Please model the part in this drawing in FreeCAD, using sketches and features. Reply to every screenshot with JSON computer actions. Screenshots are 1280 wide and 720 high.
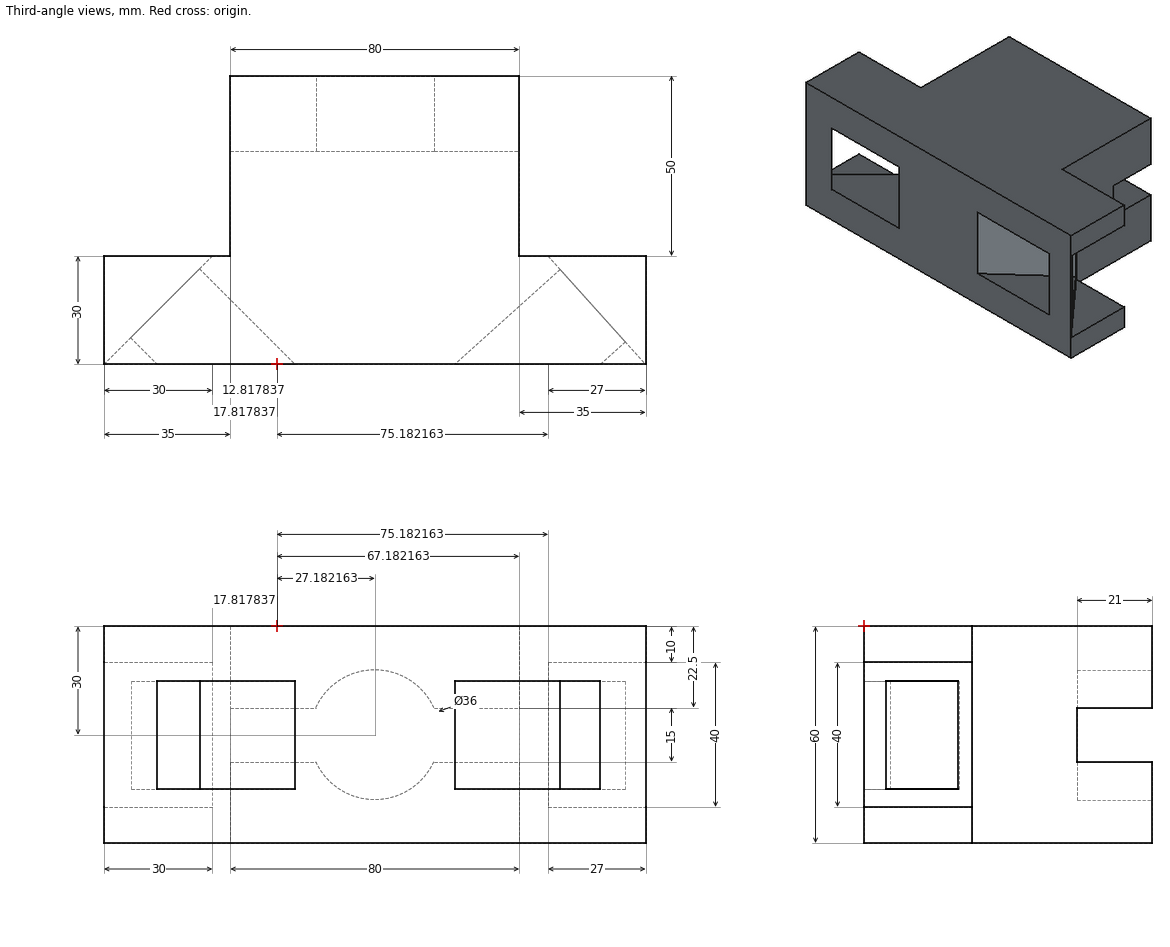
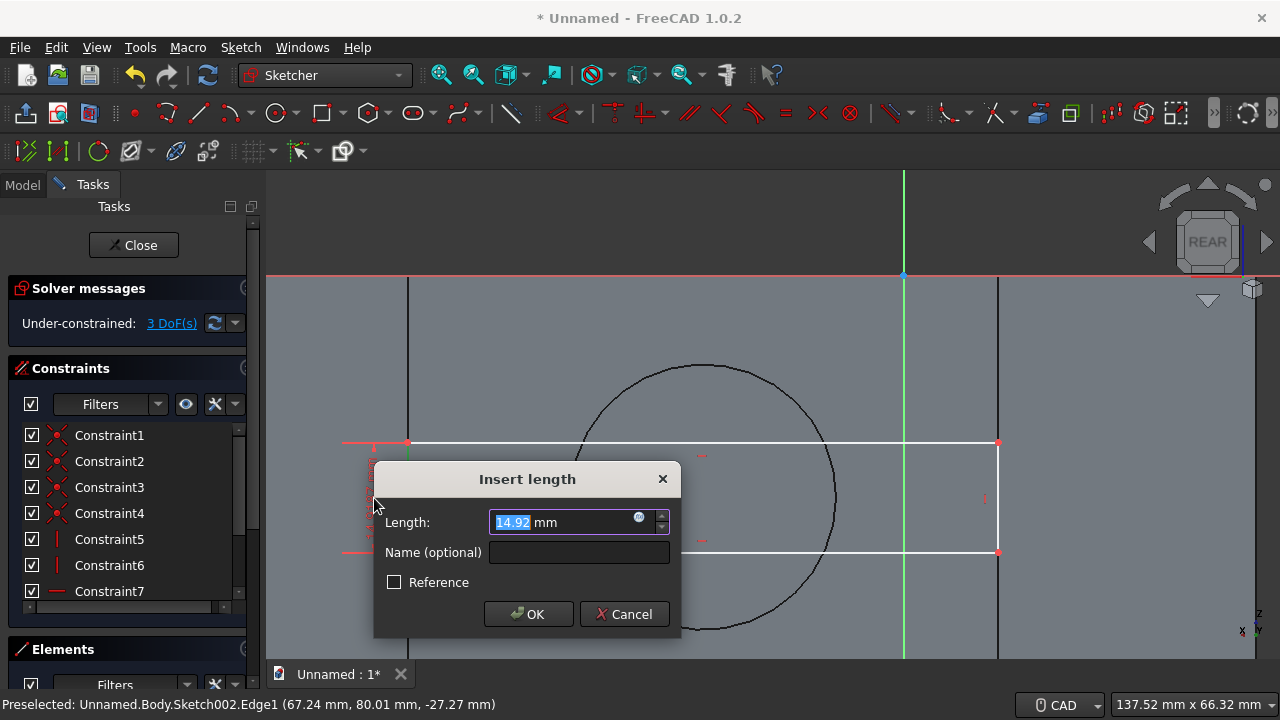
{"action": "type", "text": "15"}
{"action": "key", "text": "Return"}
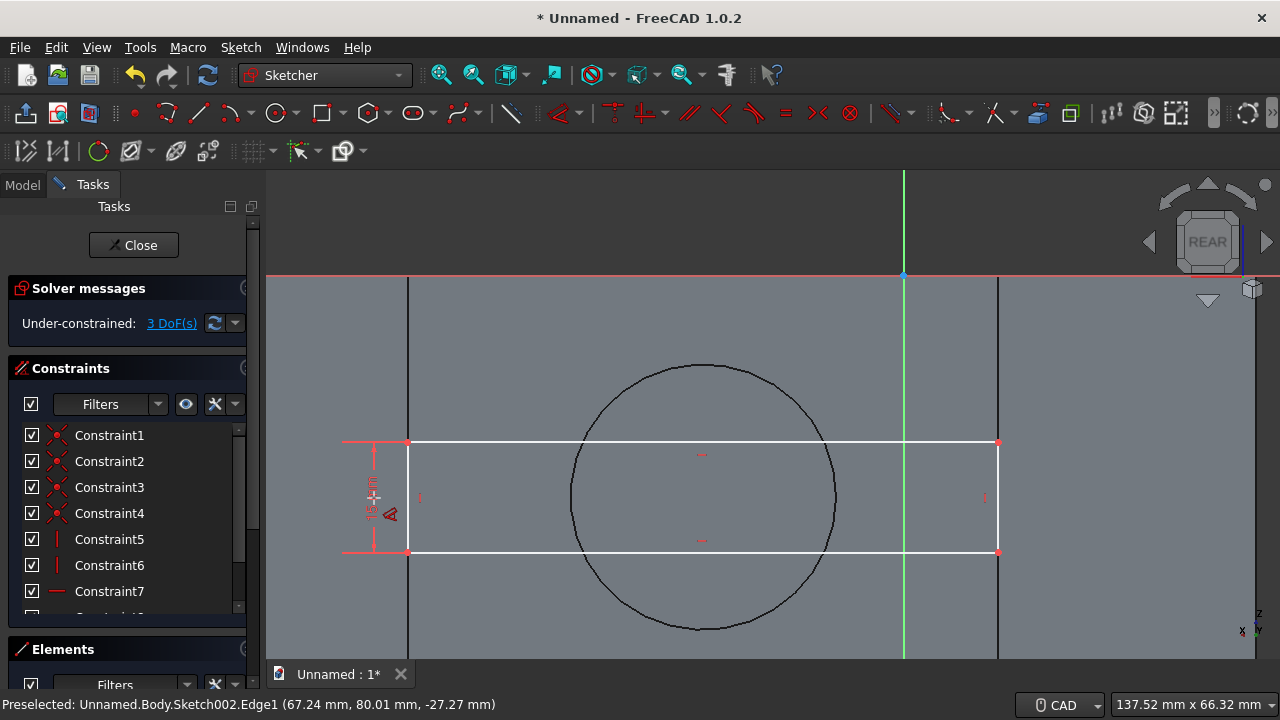
{"action": "left_click", "coordinate": [585, 553]}
{"action": "left_click", "coordinate": [703, 587]}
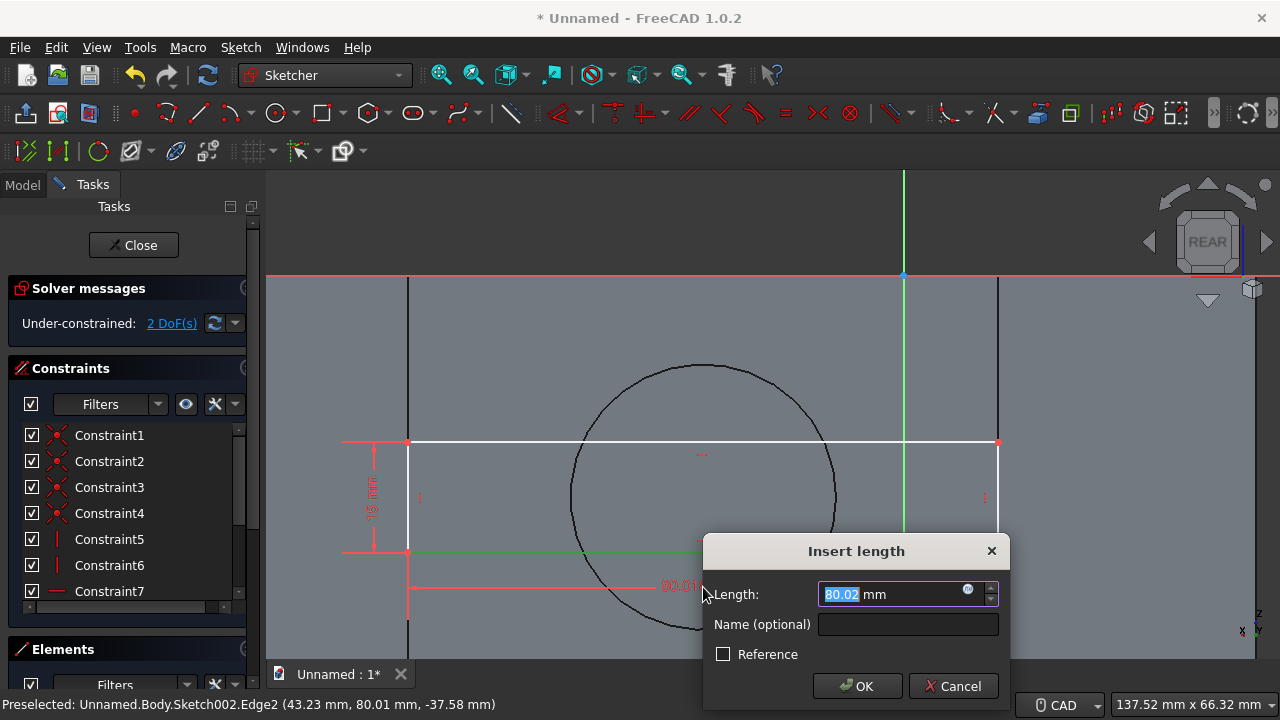
{"action": "type", "text": "80"}
{"action": "key", "text": "Return"}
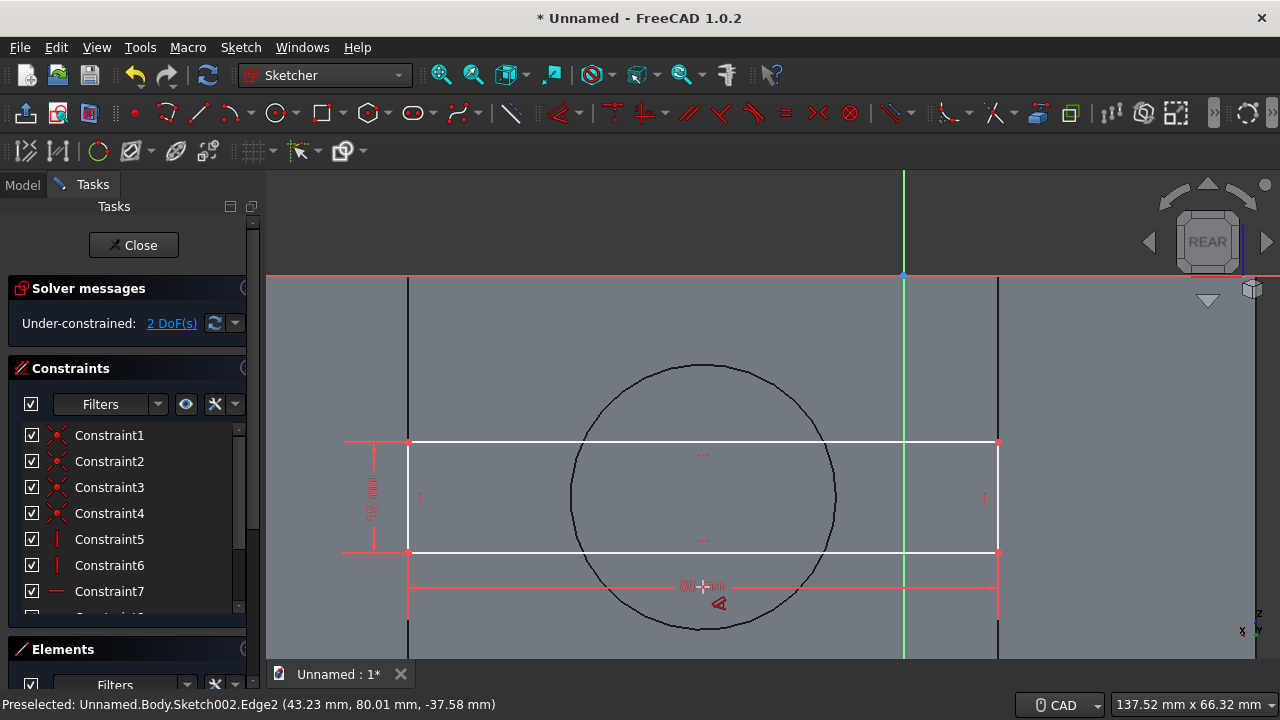
{"action": "left_click", "coordinate": [408, 442]}
{"action": "left_click", "coordinate": [374, 359]}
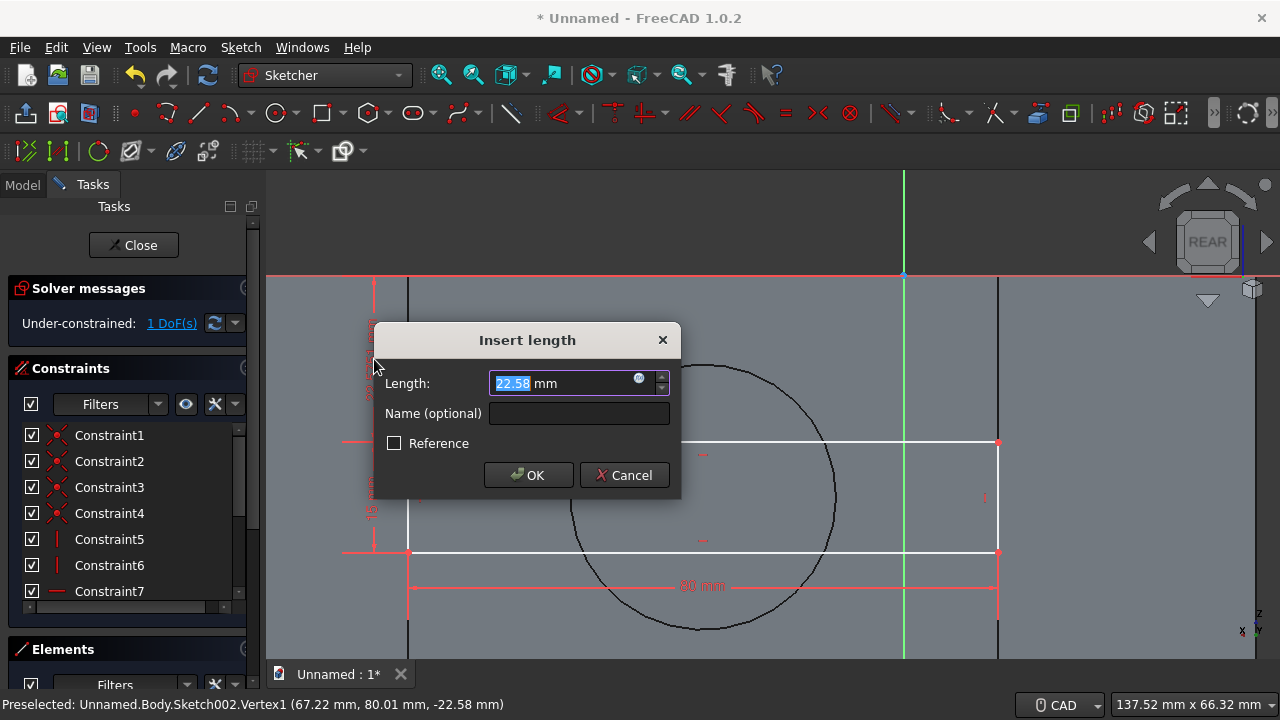
{"action": "type", "text": "22.5"}
{"action": "key", "text": "Return"}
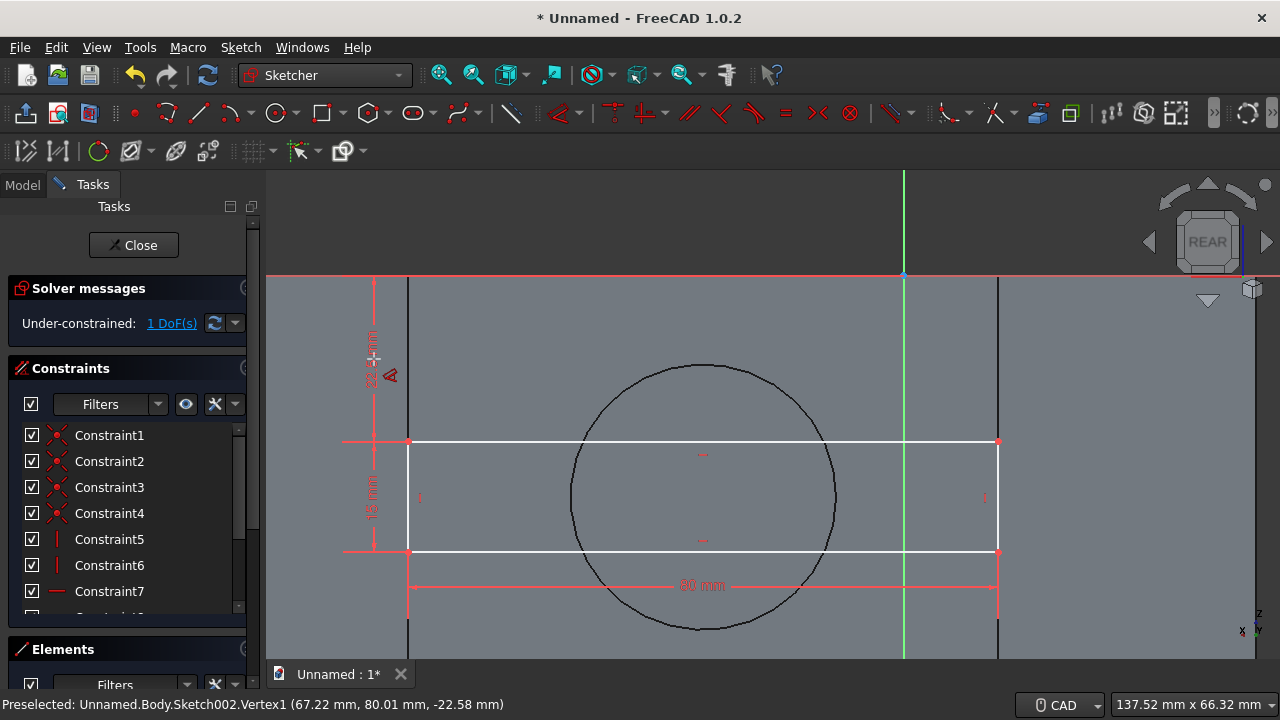
{"action": "left_click", "coordinate": [408, 442]}
{"action": "left_click", "coordinate": [656, 242]}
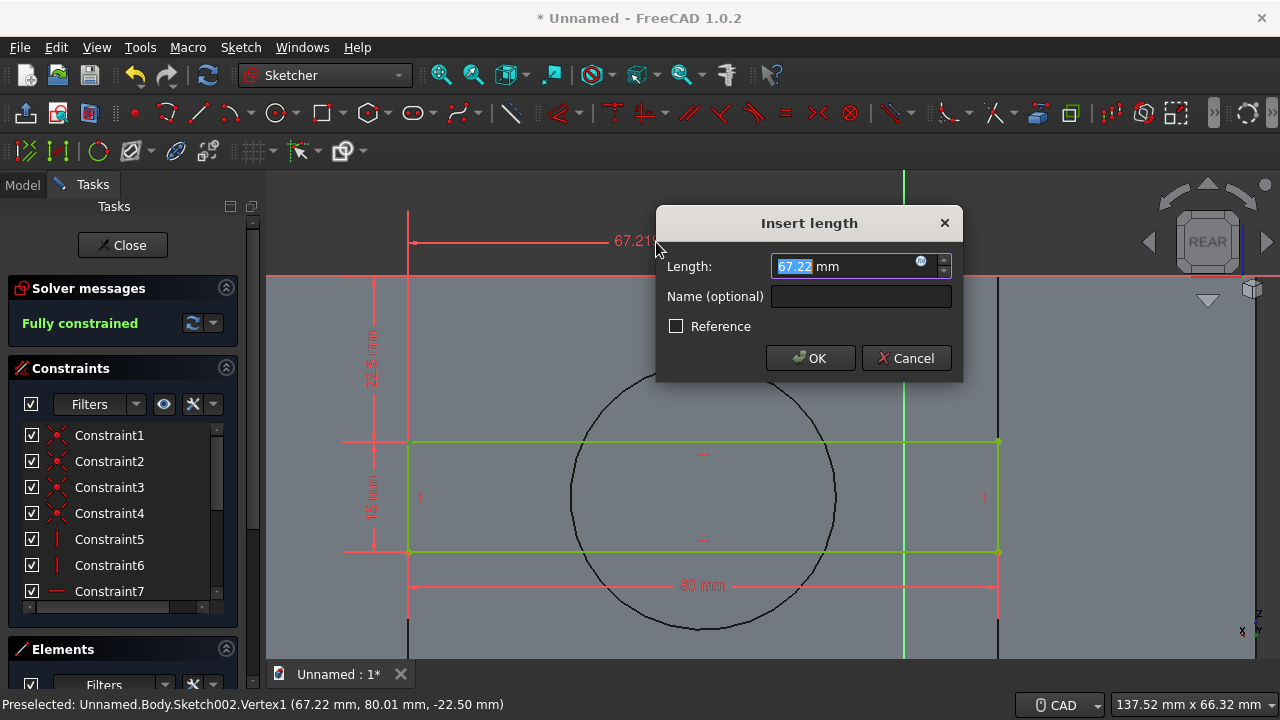
{"action": "type", "text": "67.182163"}
{"action": "key", "text": "Return"}
{"action": "key", "text": "Escape"}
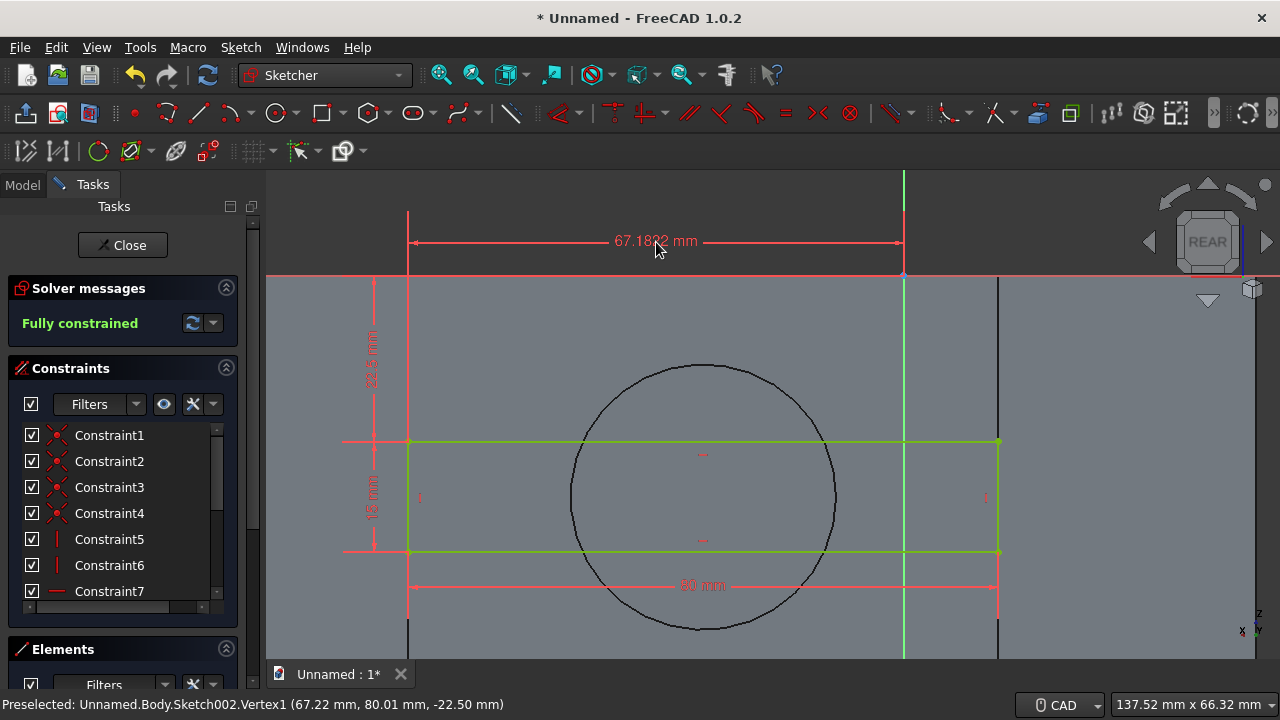
{"action": "left_click", "coordinate": [123, 245]}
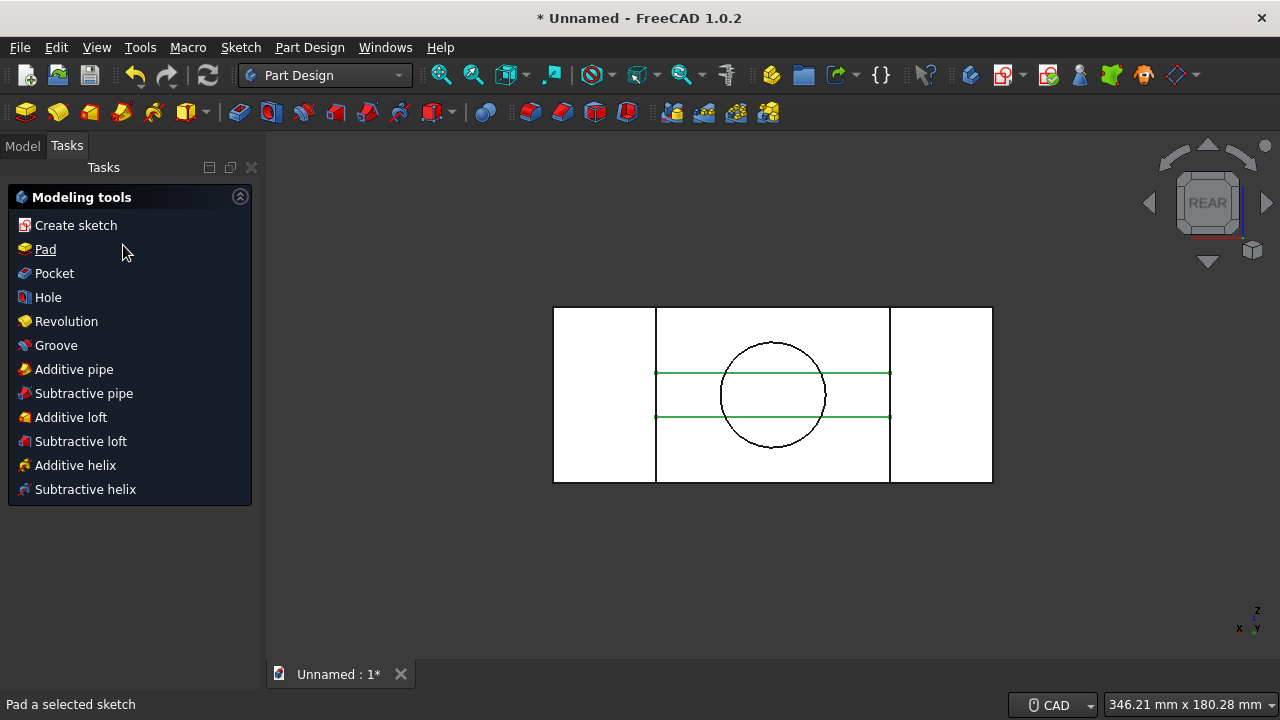
{"action": "left_click", "coordinate": [240, 112]}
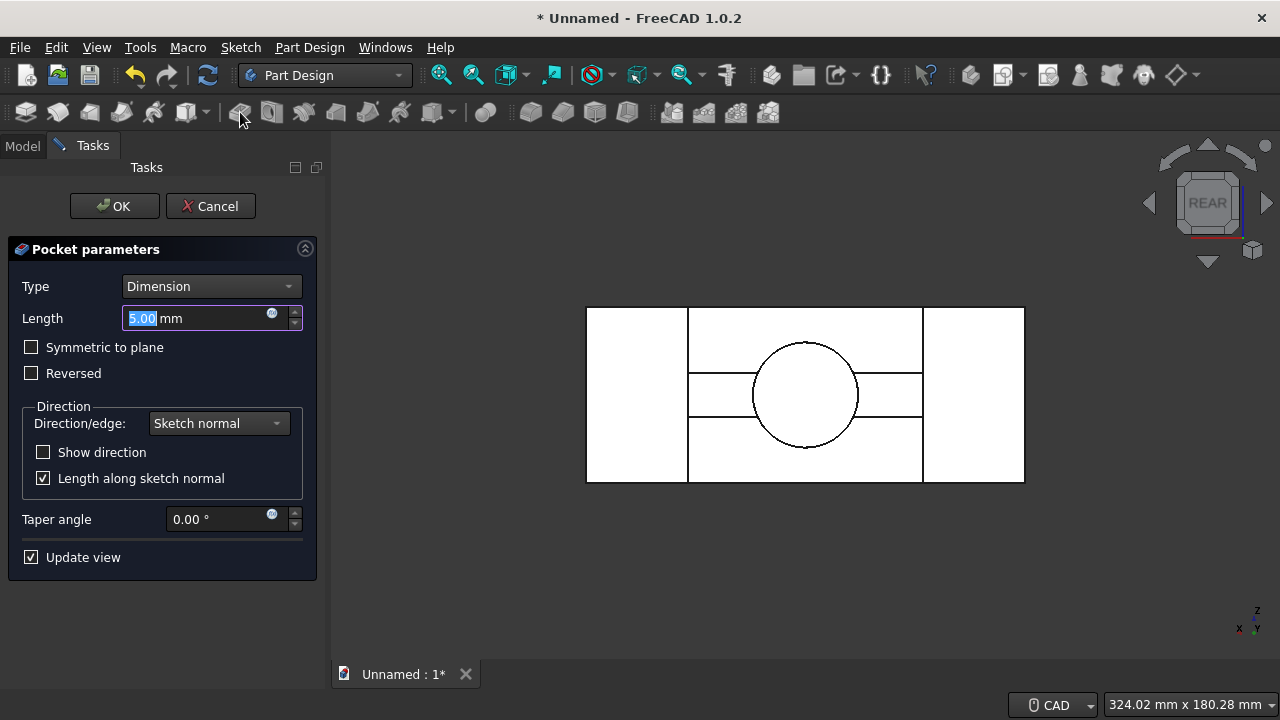
{"action": "type", "text": "21"}
{"action": "key", "text": "Tab"}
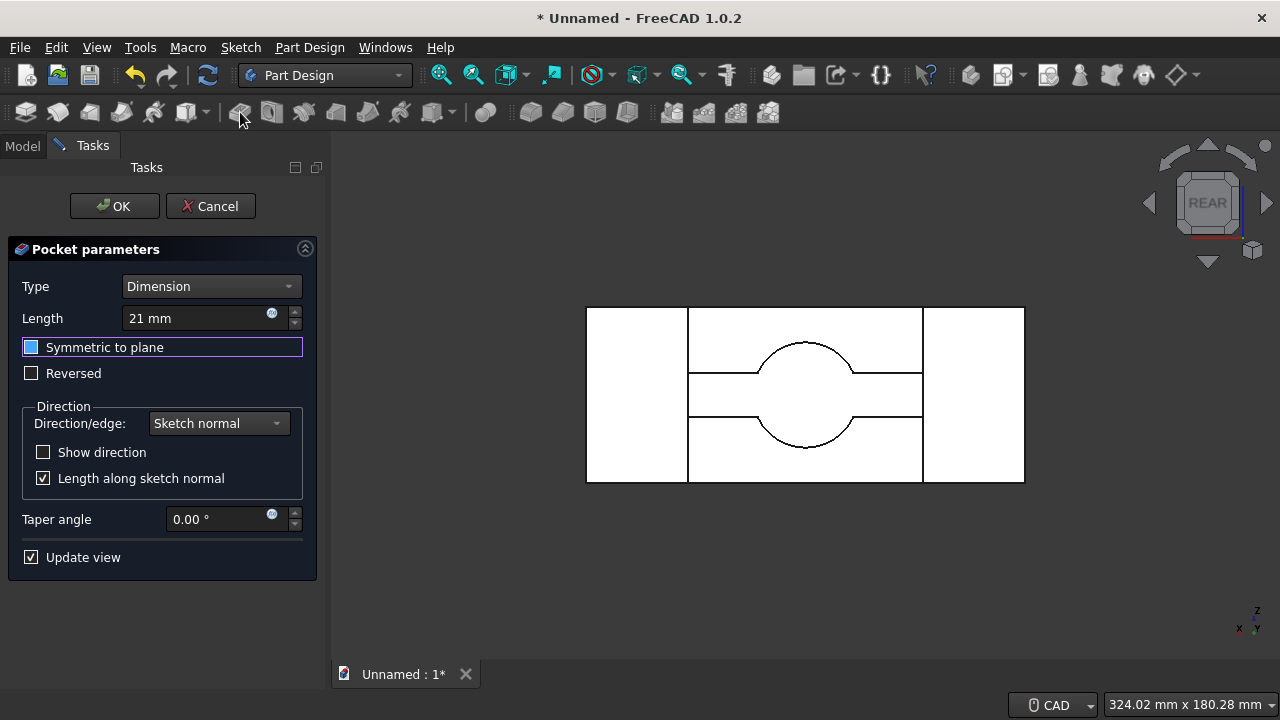
{"action": "left_click", "coordinate": [115, 206]}